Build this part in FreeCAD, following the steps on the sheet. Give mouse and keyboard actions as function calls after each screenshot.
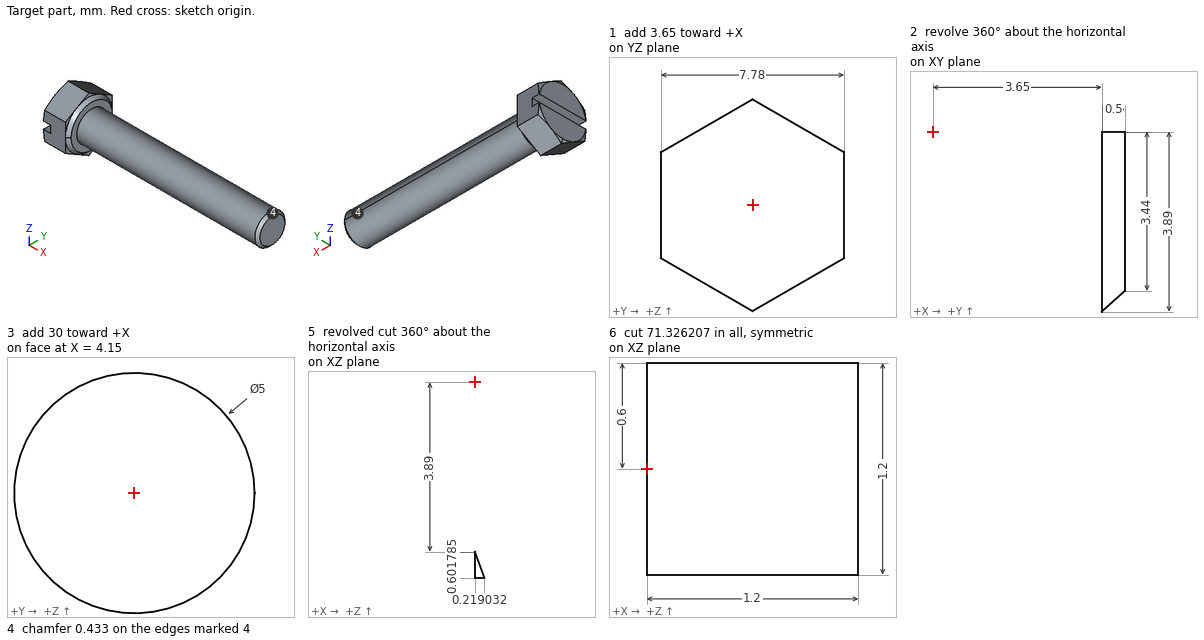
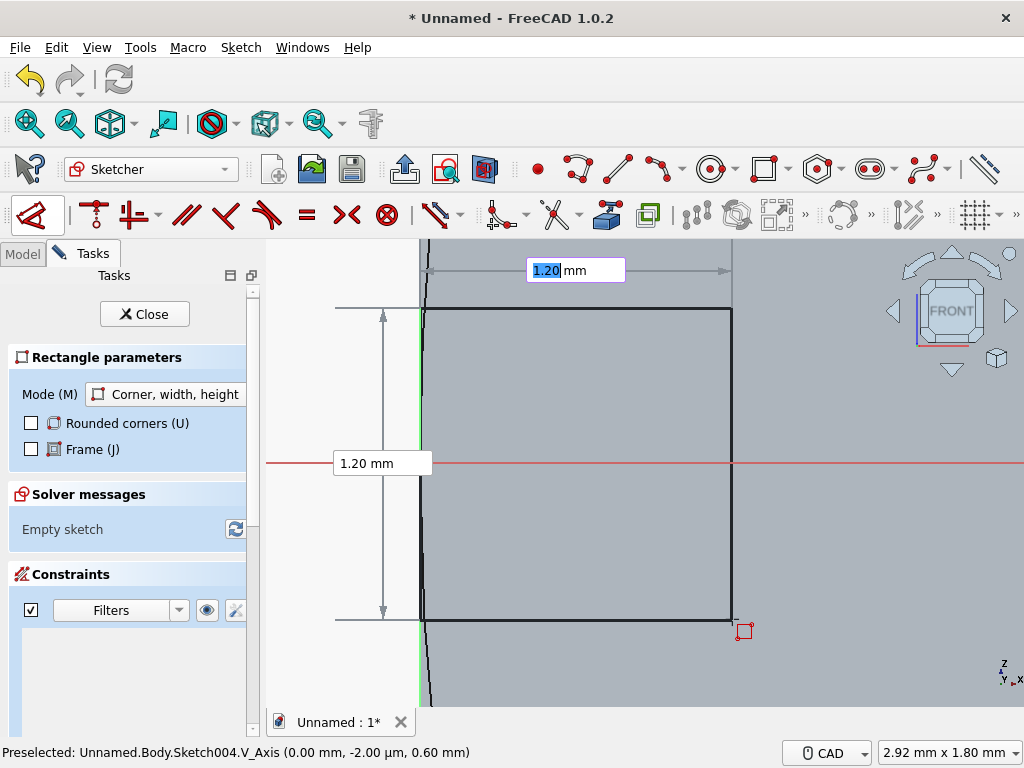
text(1.2)
key(Tab)
text(1.2)
key(Return)
key(Escape)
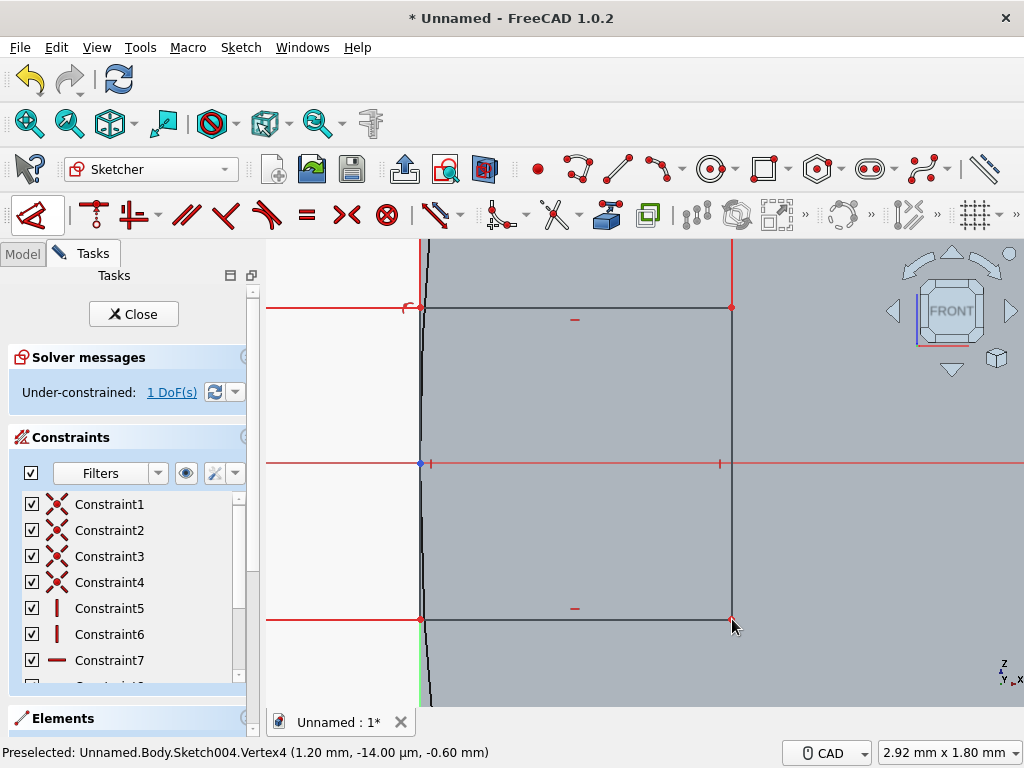
click(420, 308)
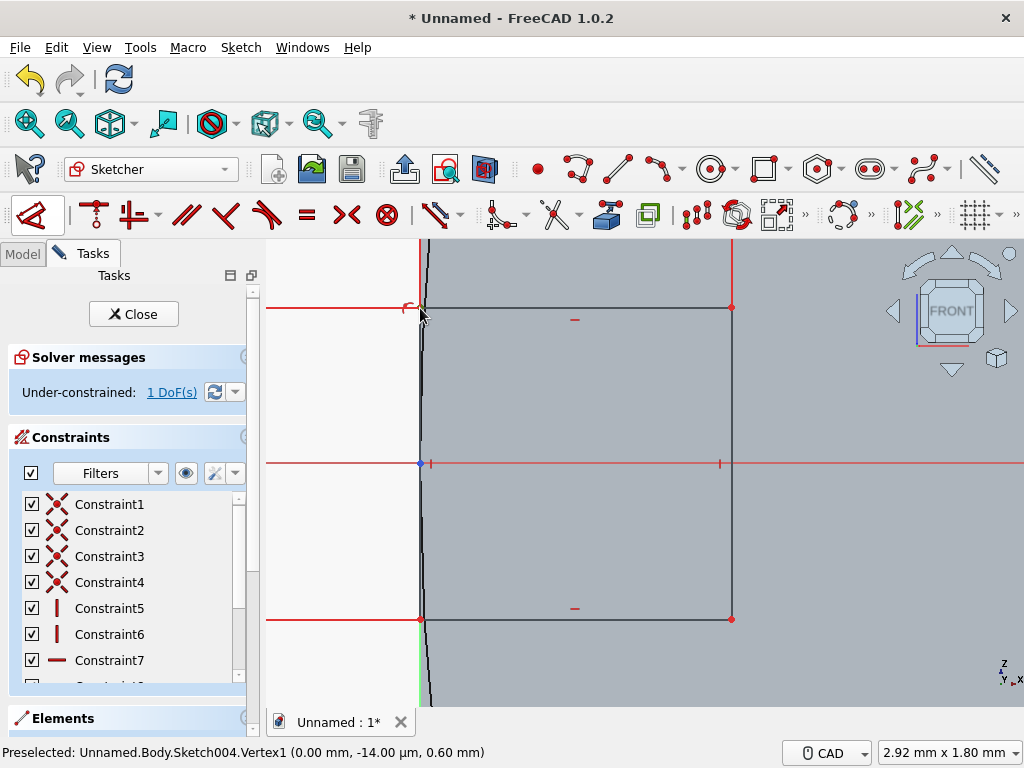
click(58, 216)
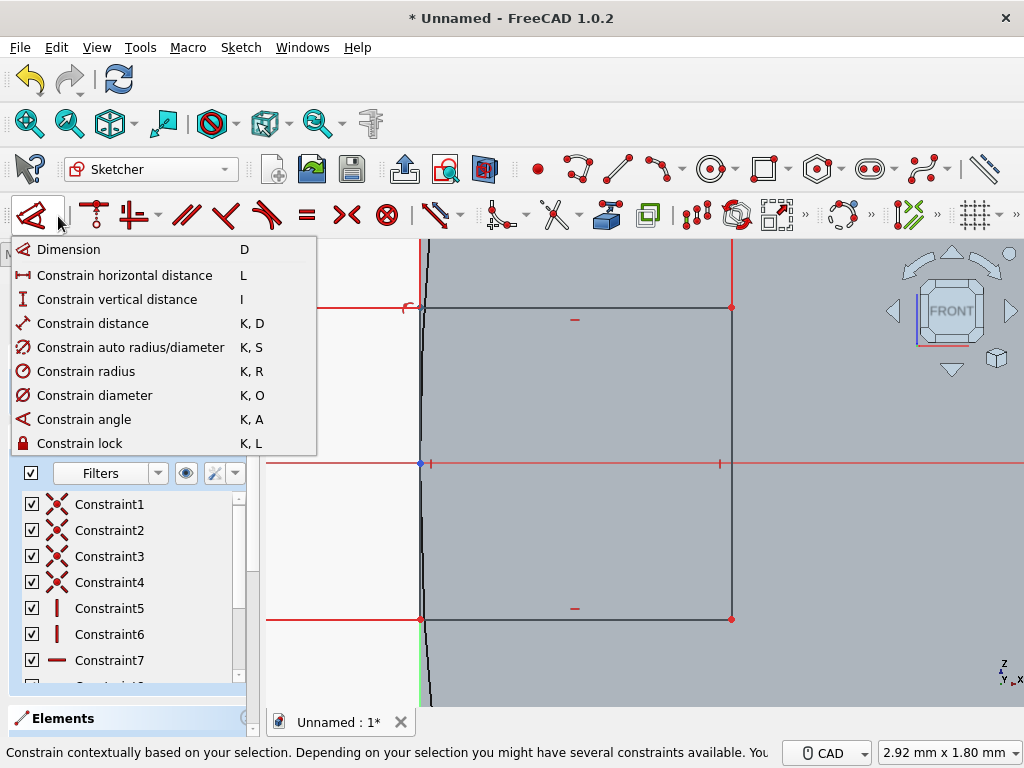
click(164, 299)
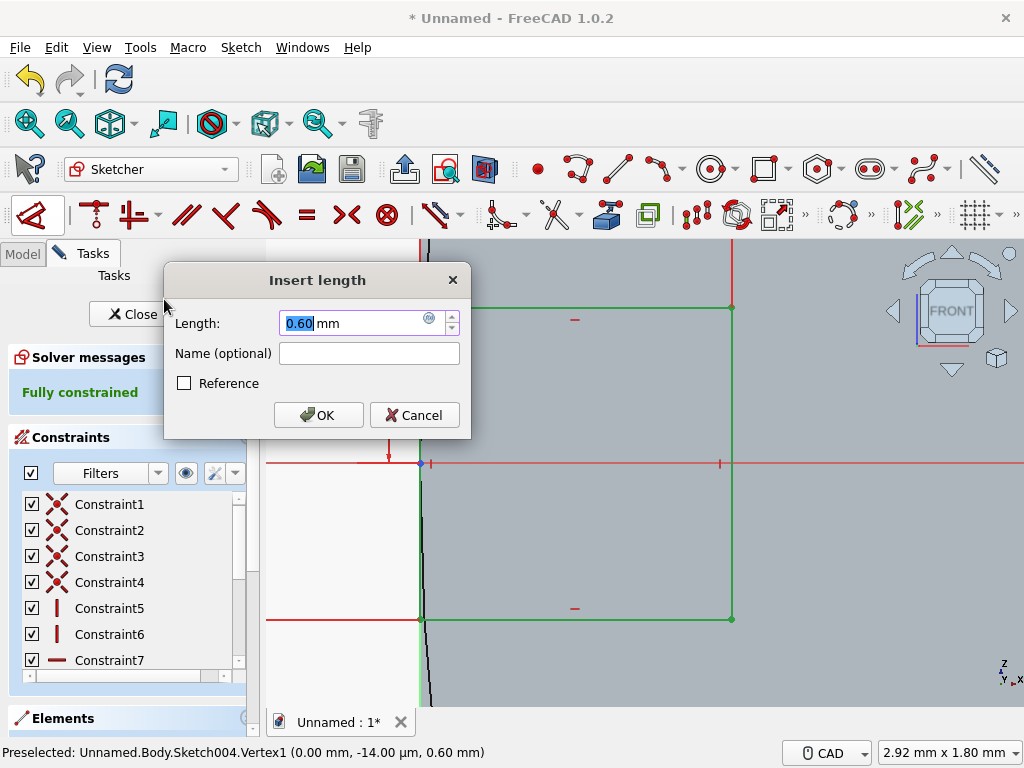
text(0.6)
key(Return)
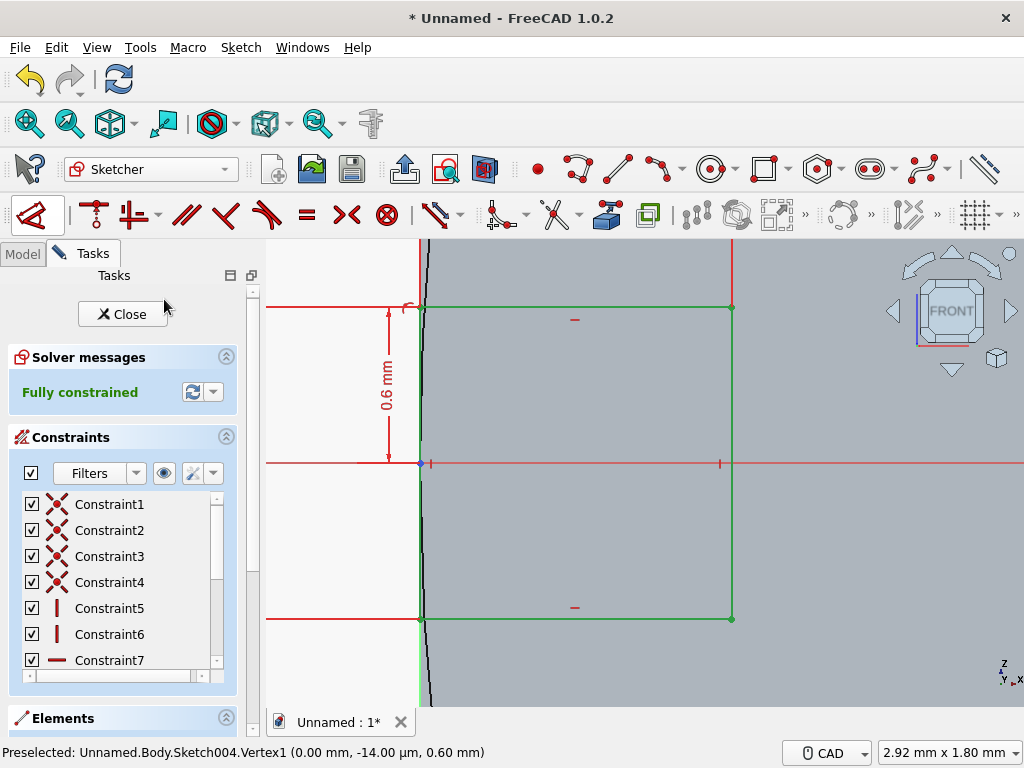
click(123, 314)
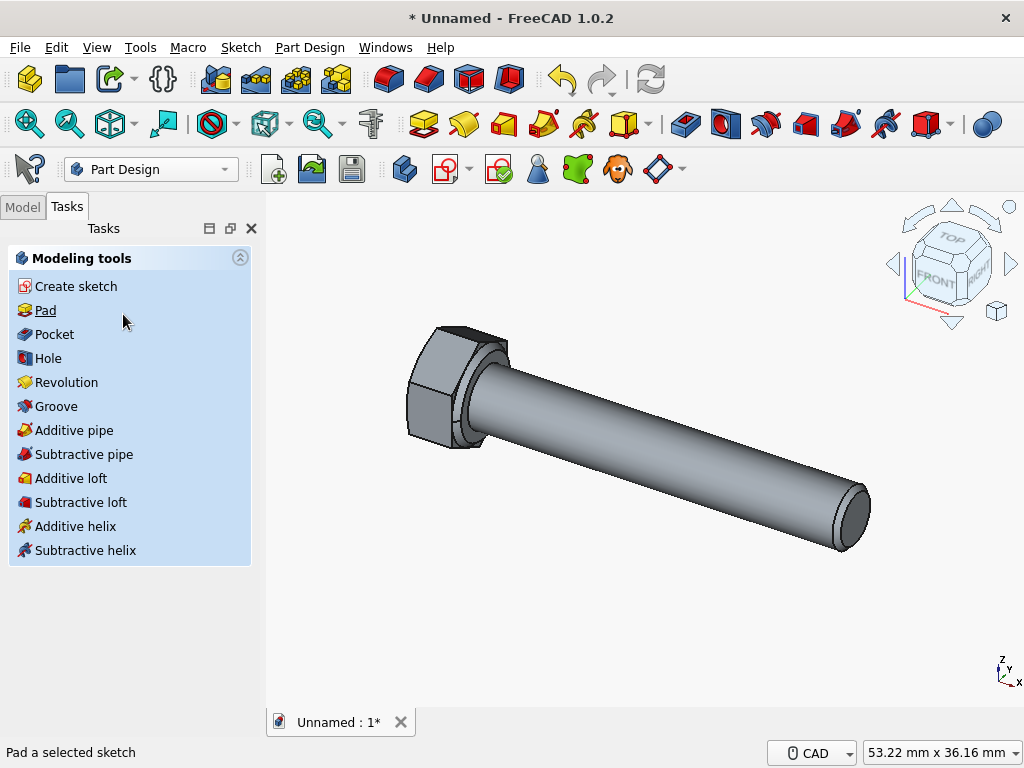
click(686, 124)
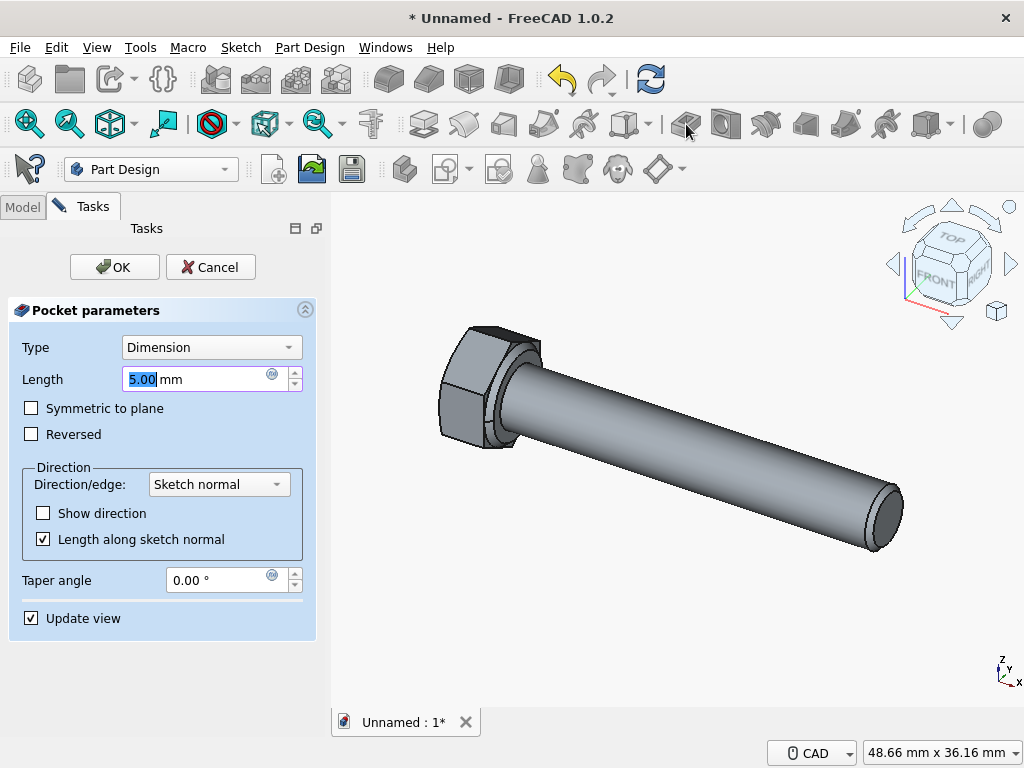
text(71.326207)
key(Tab)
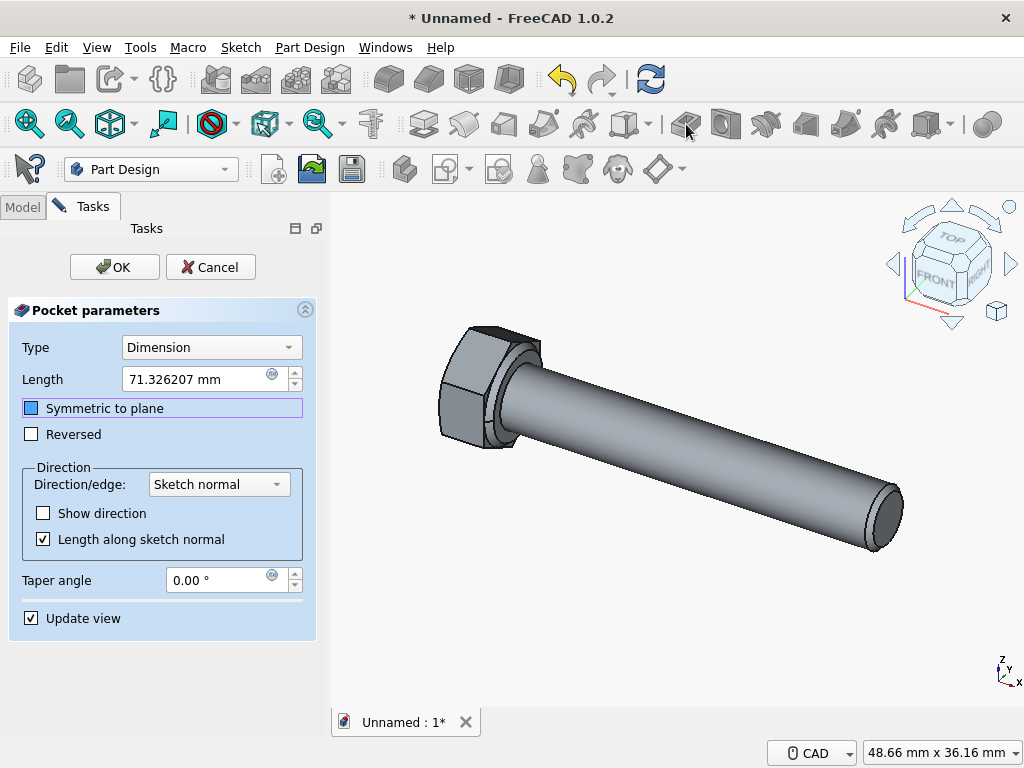
click(30, 408)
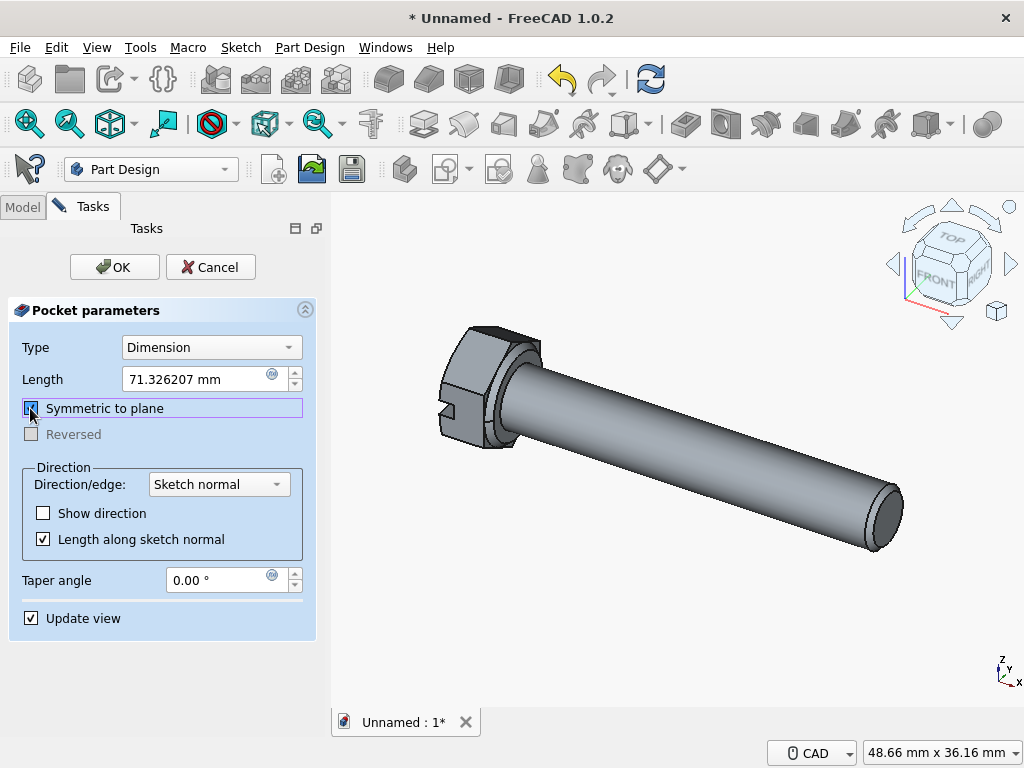
click(115, 267)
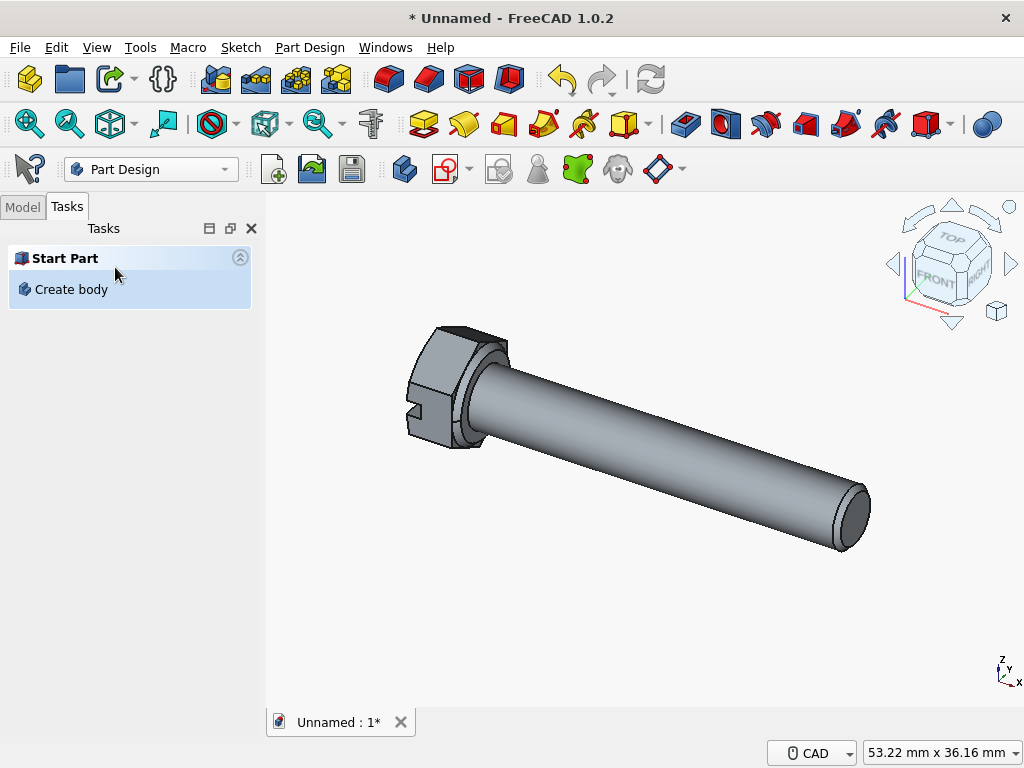
key(0)